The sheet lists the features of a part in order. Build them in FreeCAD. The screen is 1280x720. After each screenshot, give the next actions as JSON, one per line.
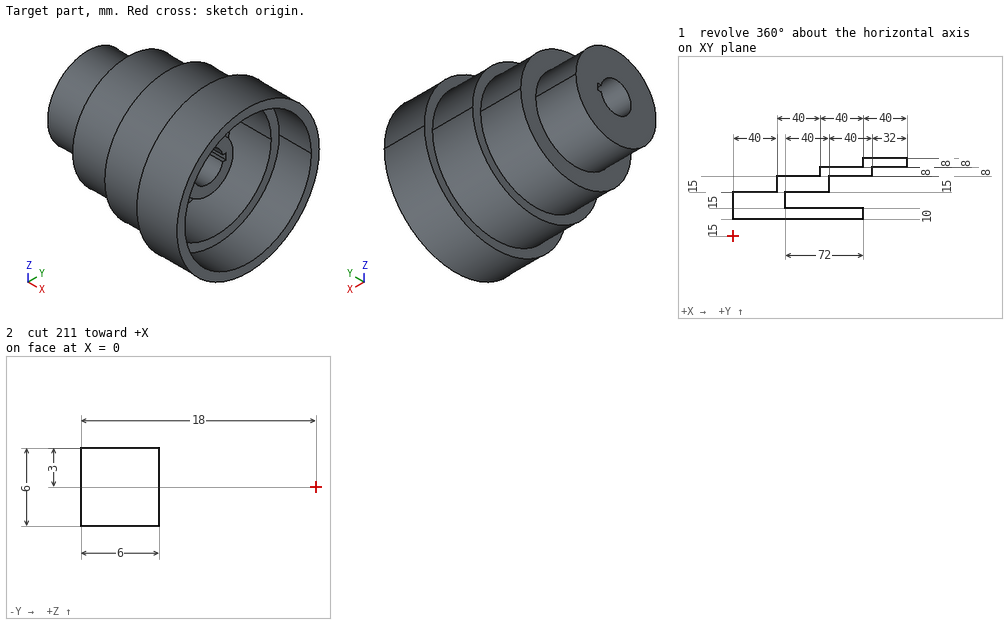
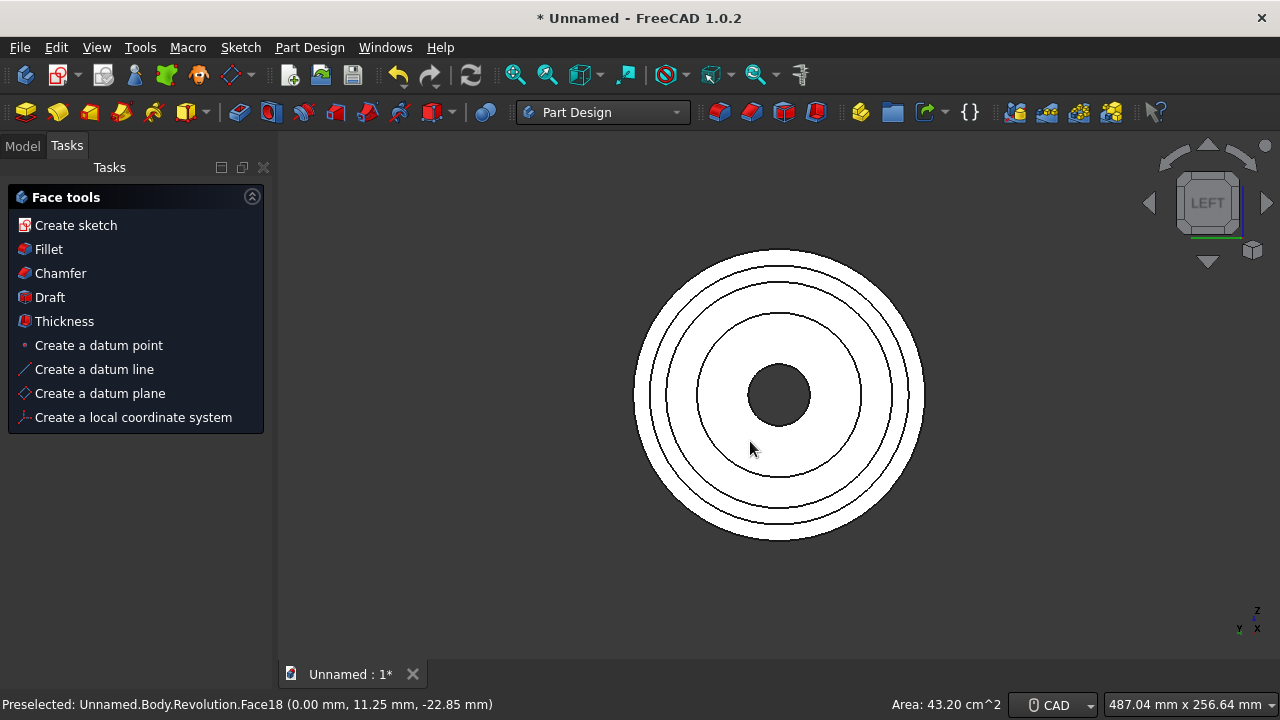
{"action": "left_click", "coordinate": [58, 76]}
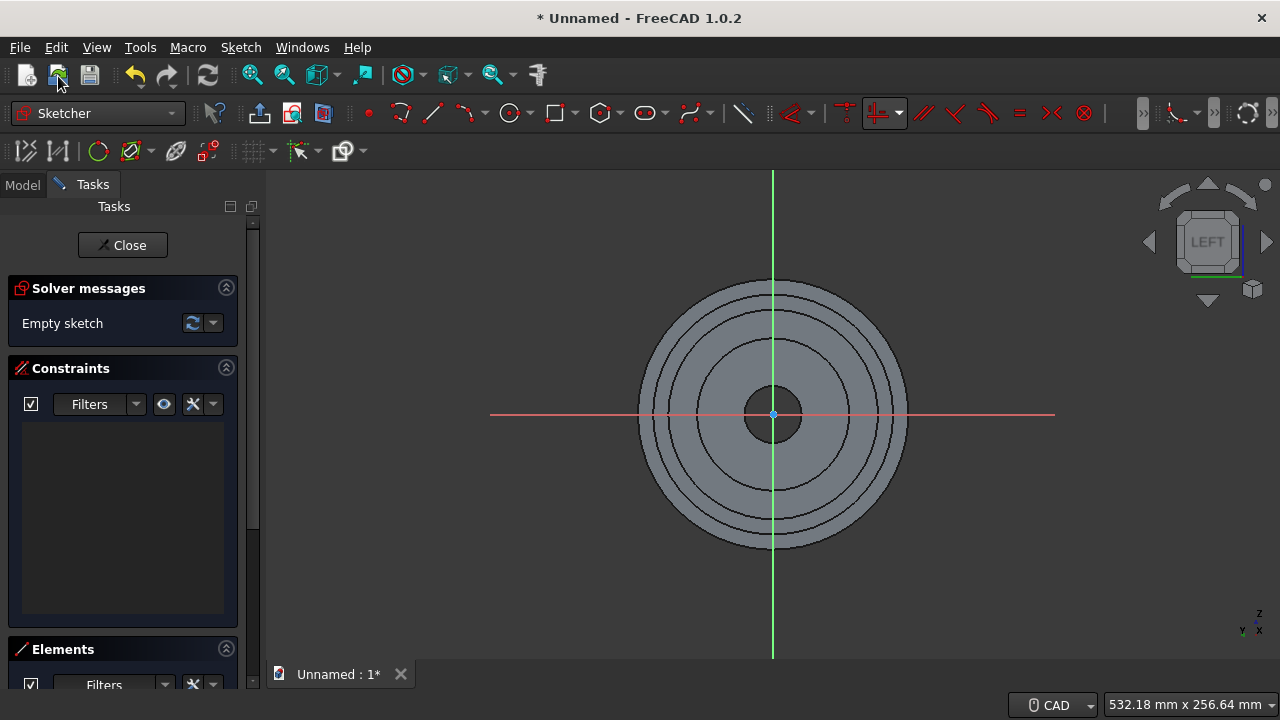
{"action": "scroll", "coordinate": [747, 414], "scroll_direction": "up", "scroll_amount": 15}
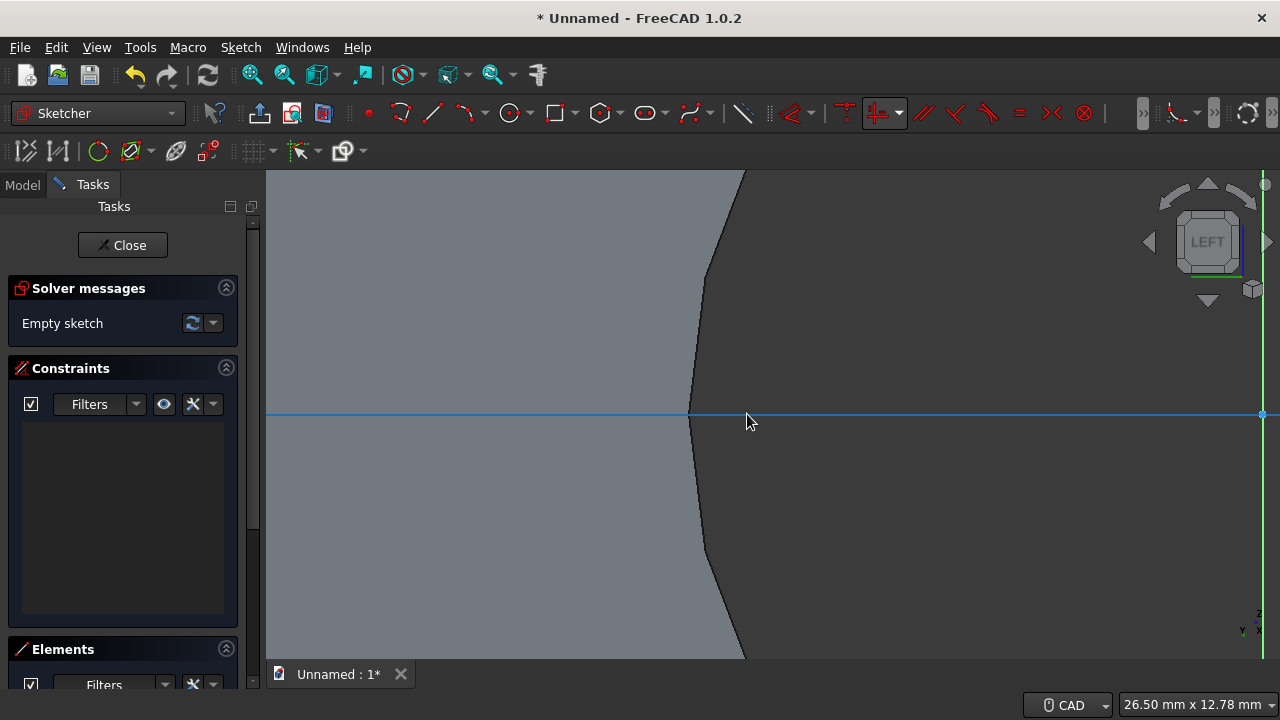
{"action": "key", "text": "g r"}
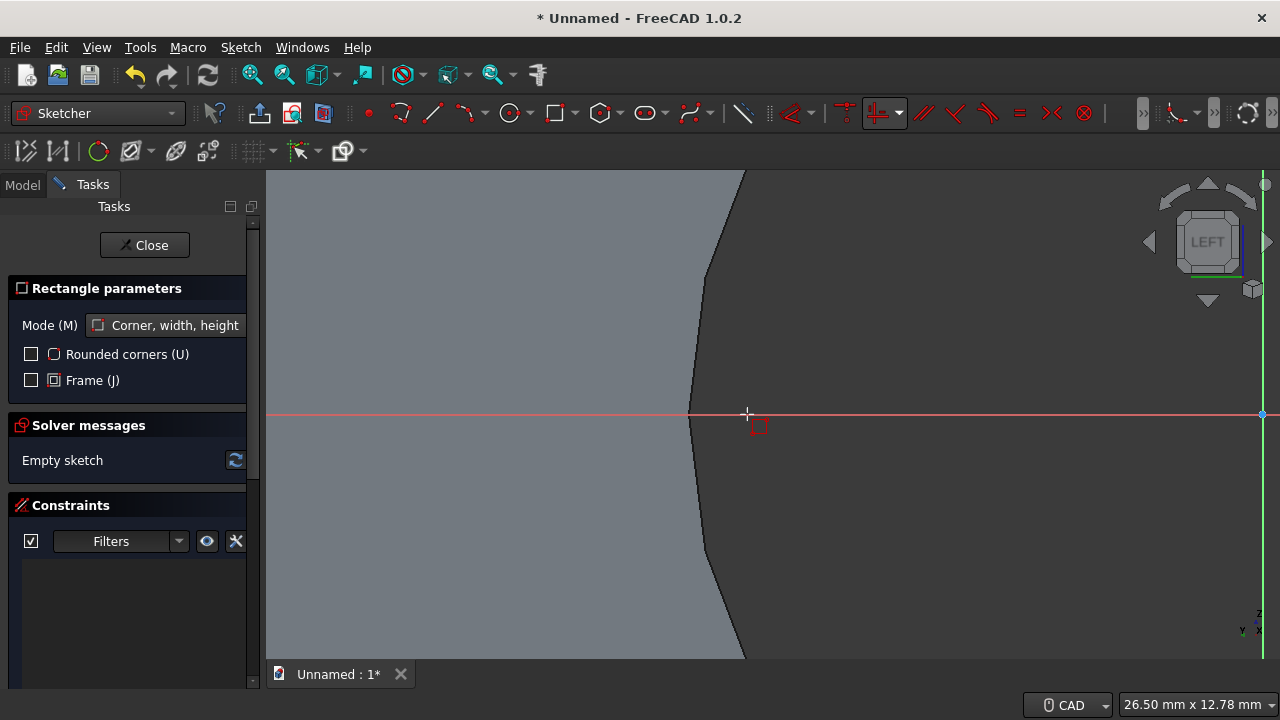
{"action": "left_click", "coordinate": [574, 300]}
{"action": "mouse_move", "coordinate": [804, 529]}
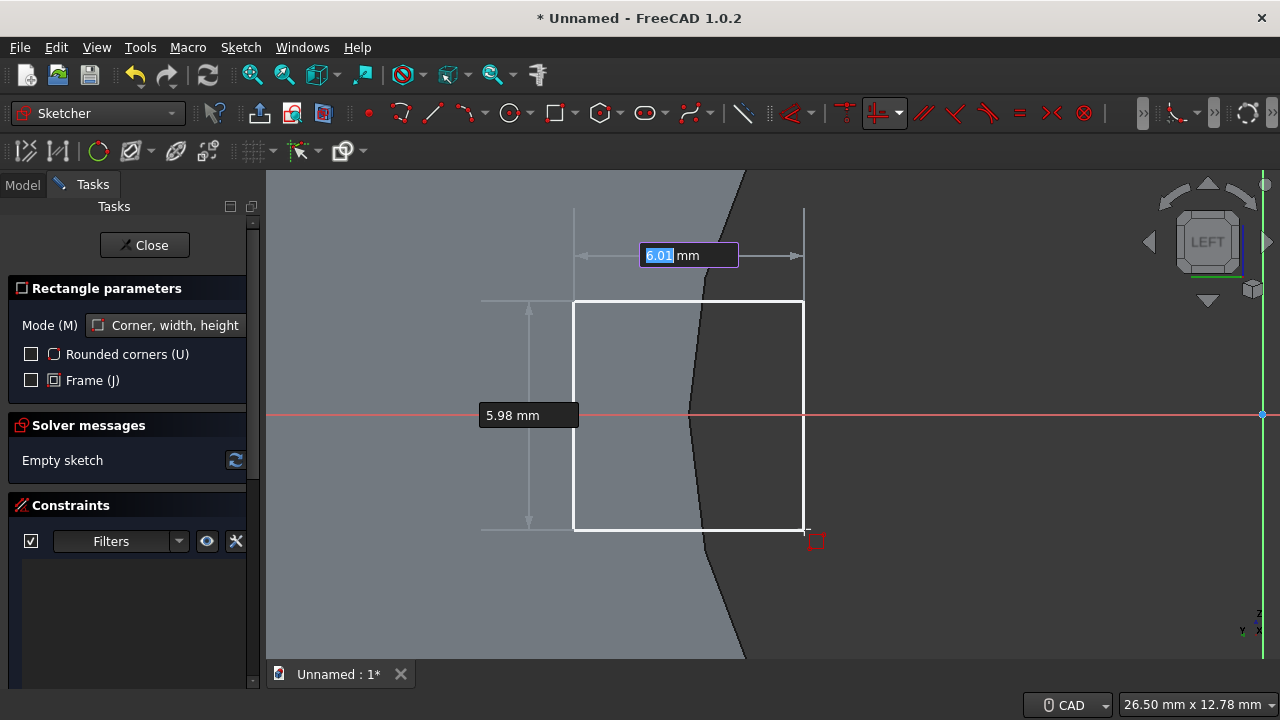
{"action": "type", "text": "6"}
{"action": "key", "text": "Tab"}
{"action": "type", "text": "6"}
{"action": "key", "text": "Return"}
{"action": "key", "text": "Escape"}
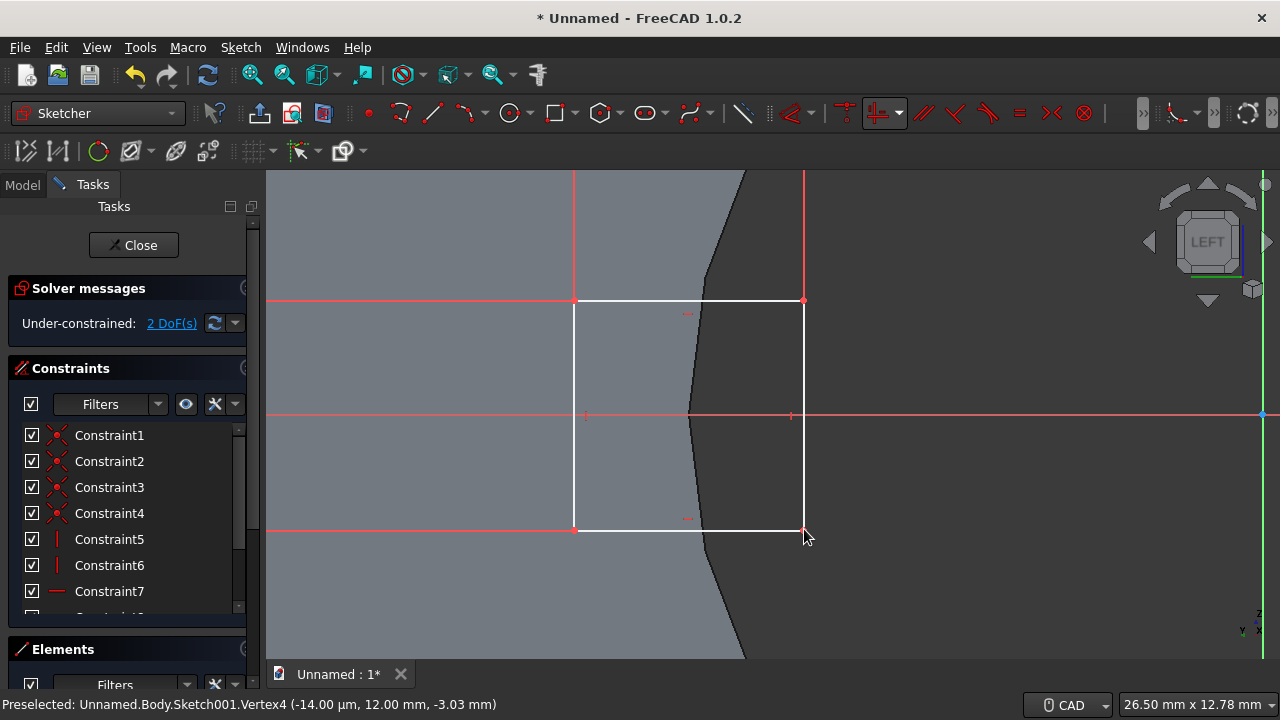
{"action": "key", "text": "d"}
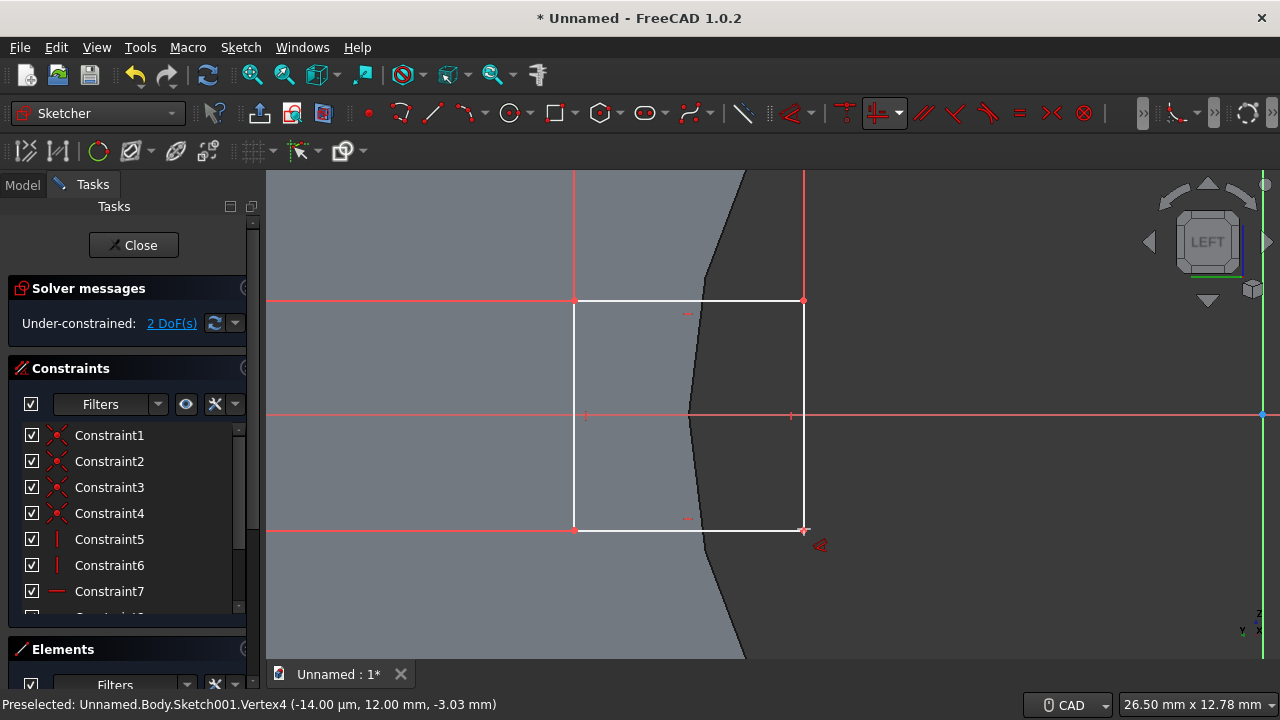
{"action": "left_click", "coordinate": [574, 301]}
{"action": "left_click", "coordinate": [540, 358]}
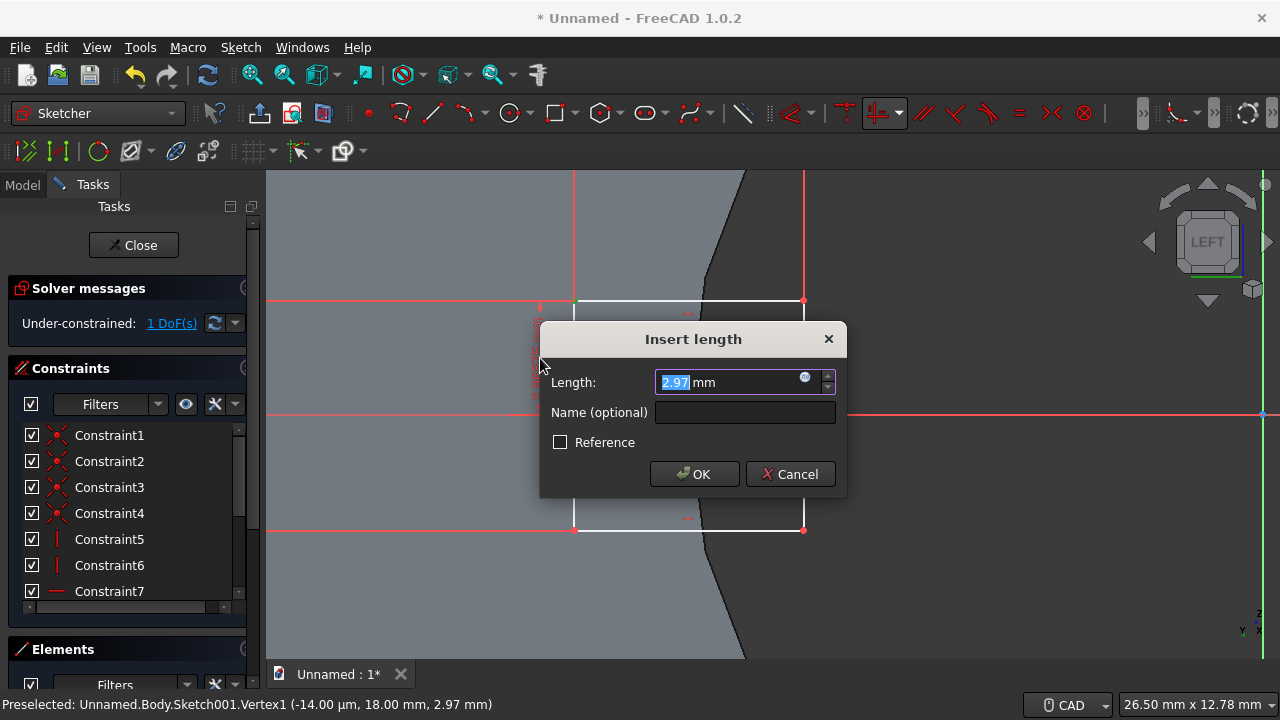
{"action": "type", "text": "3"}
{"action": "key", "text": "Return"}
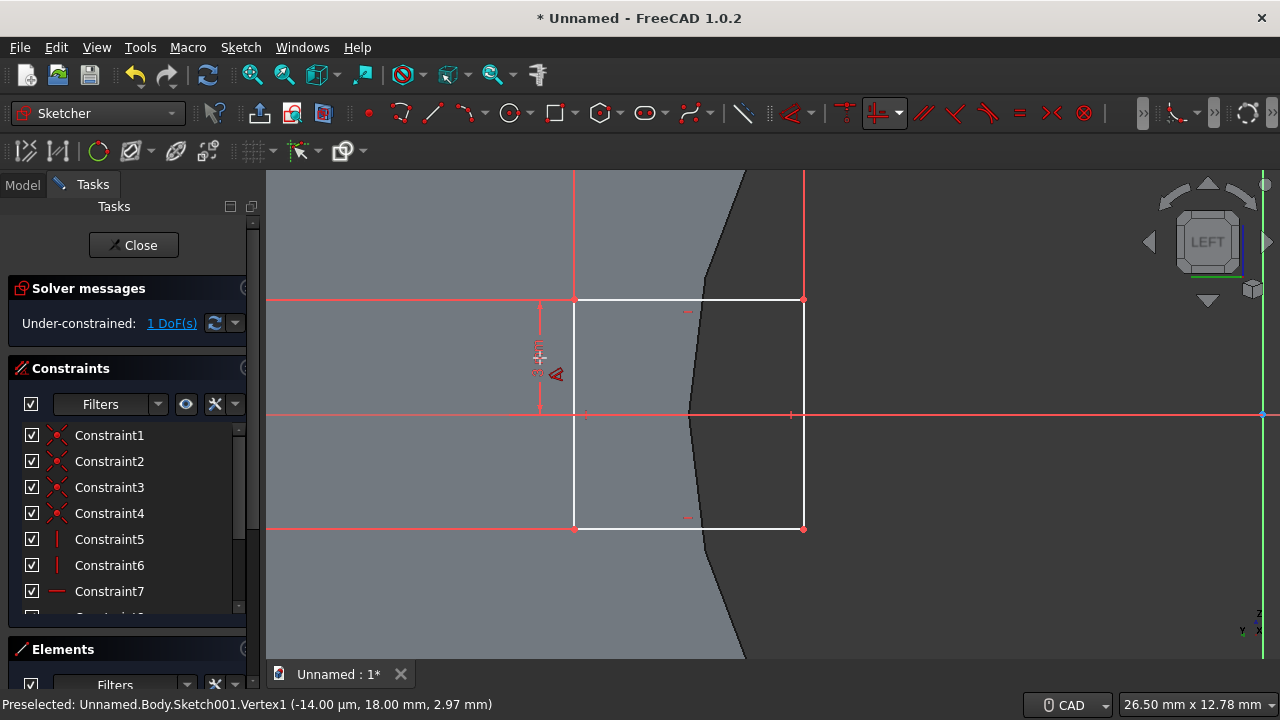
{"action": "left_click", "coordinate": [574, 300]}
{"action": "left_click", "coordinate": [845, 266]}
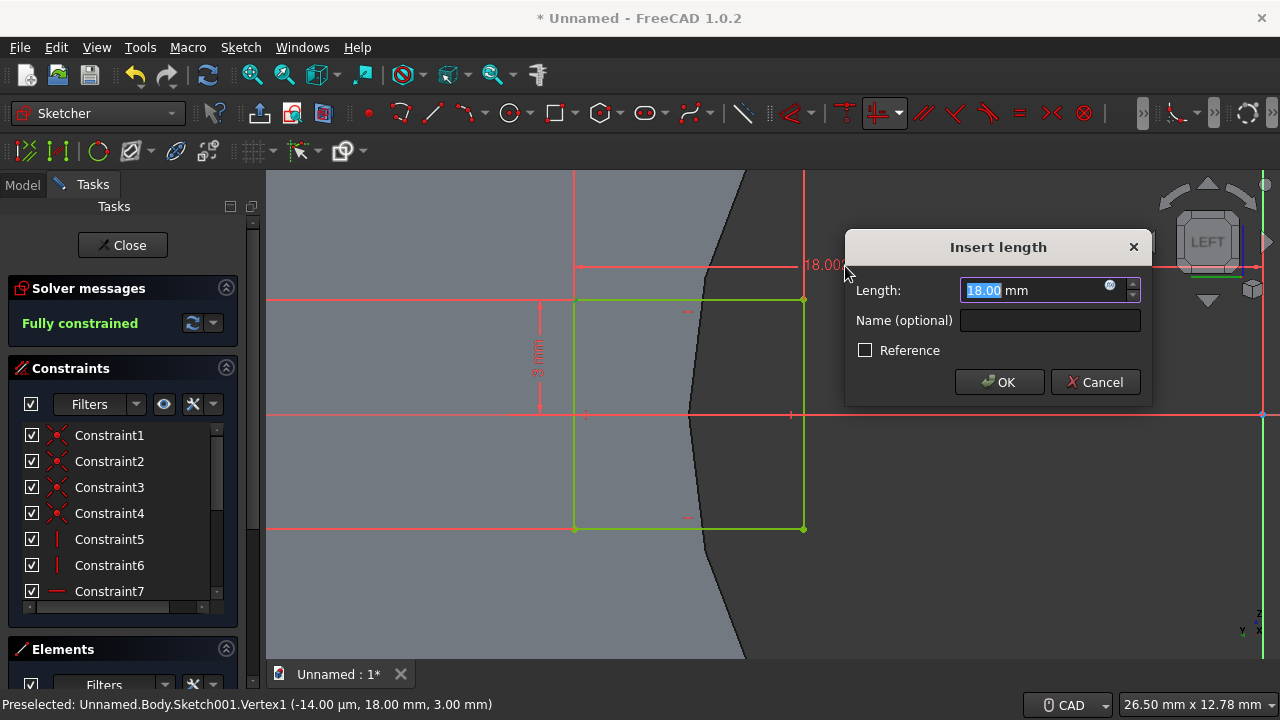
{"action": "type", "text": "18"}
{"action": "key", "text": "Return"}
{"action": "key", "text": "Escape"}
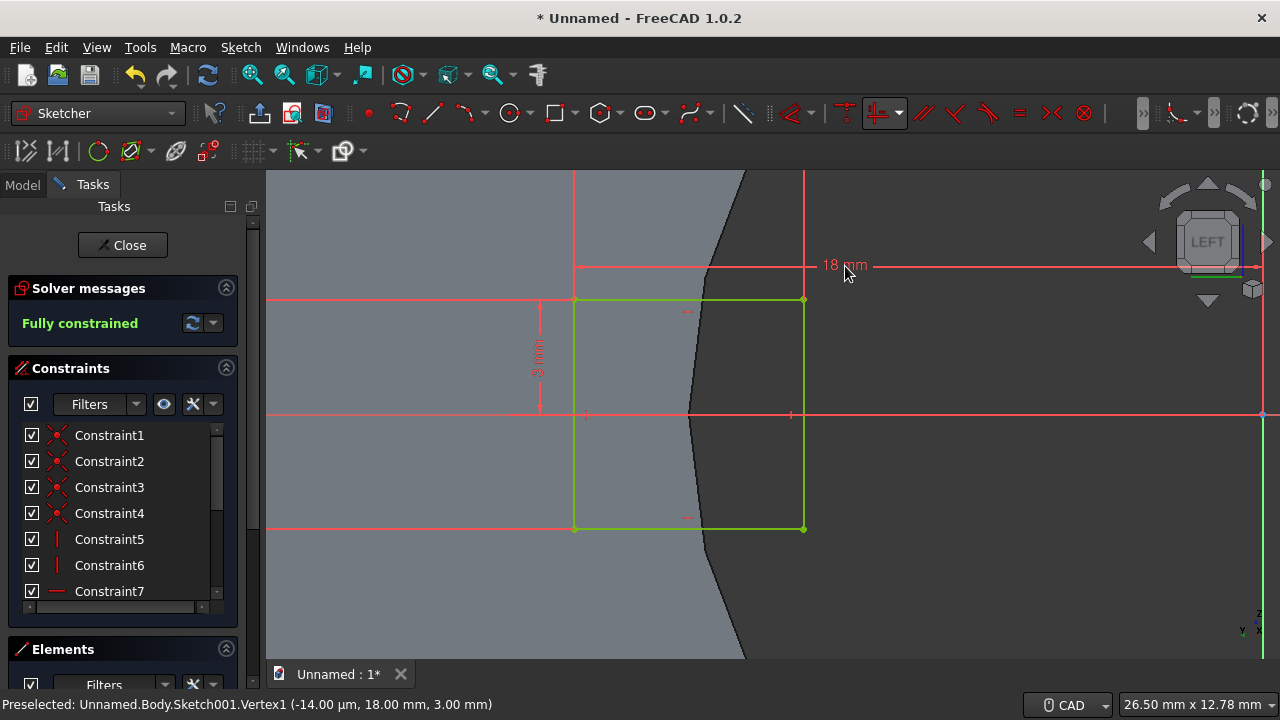
{"action": "left_click", "coordinate": [123, 245]}